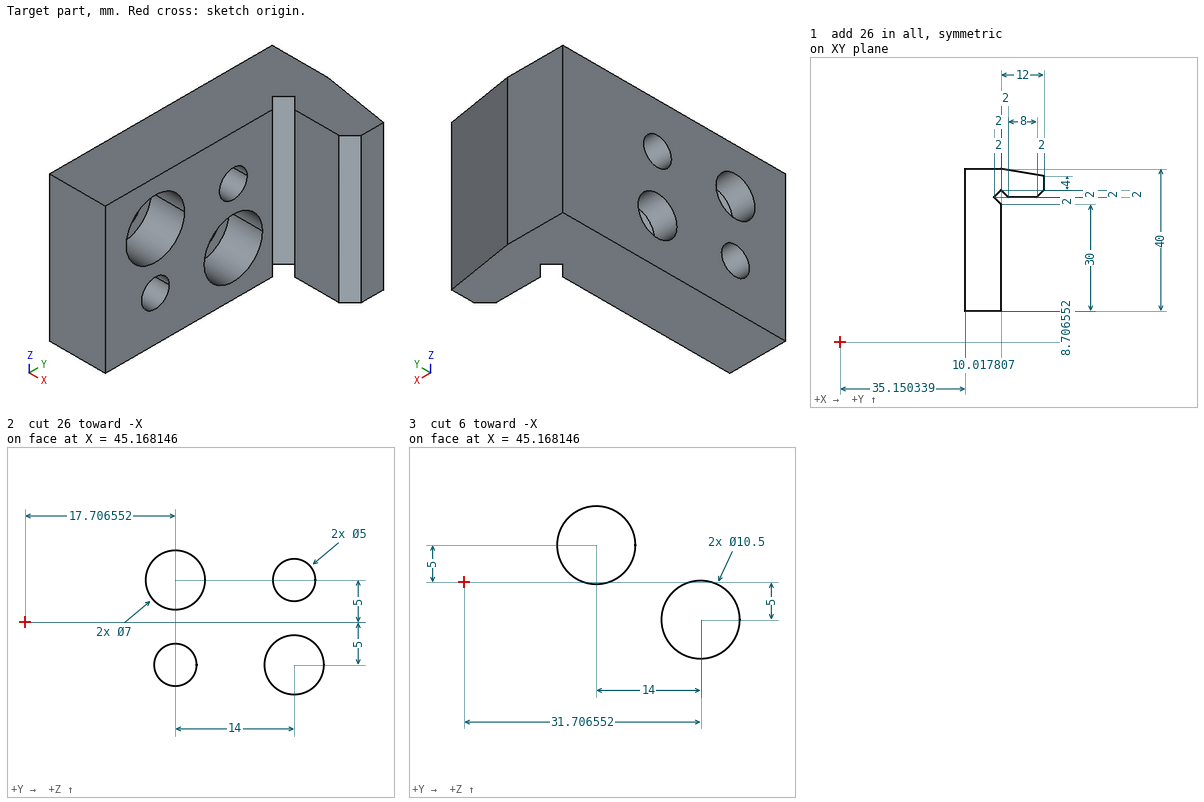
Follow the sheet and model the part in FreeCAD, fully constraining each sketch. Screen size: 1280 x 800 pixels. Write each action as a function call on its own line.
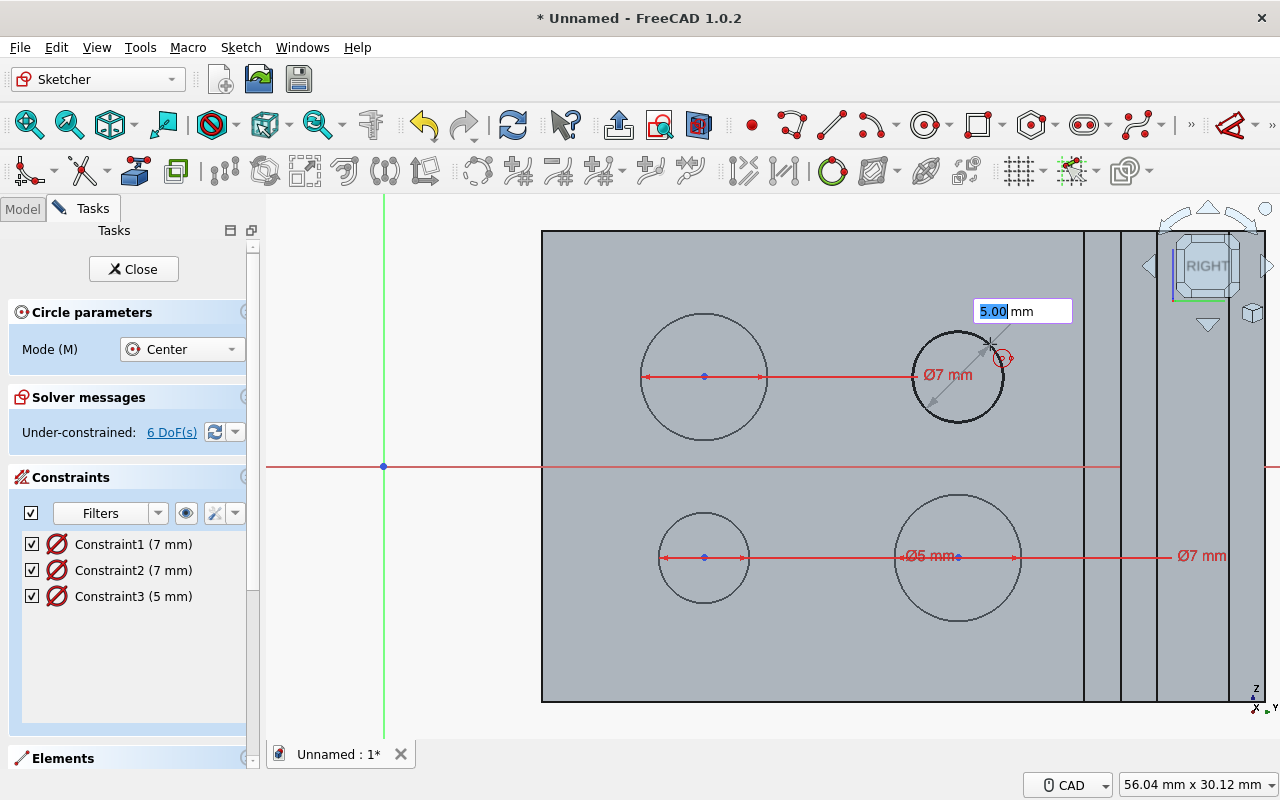
text(5)
key(Return)
key(Escape)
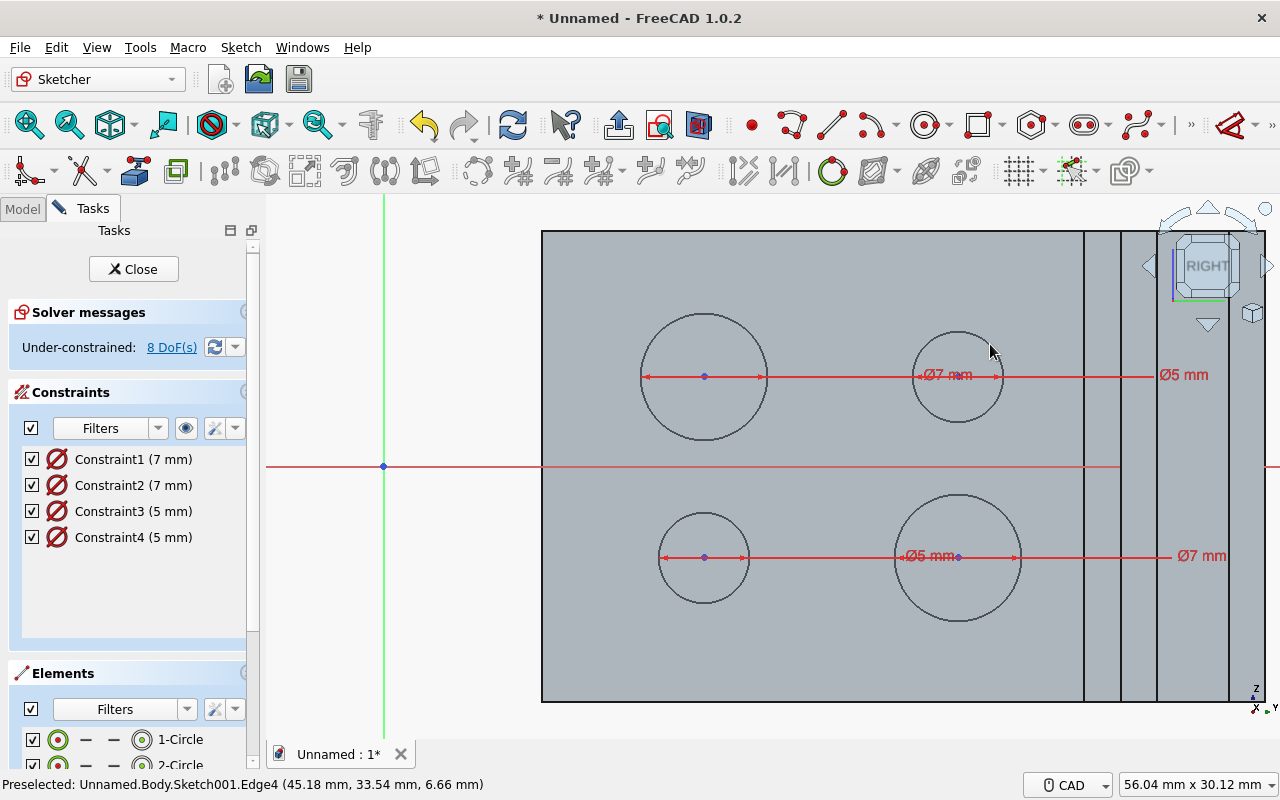
click(704, 377)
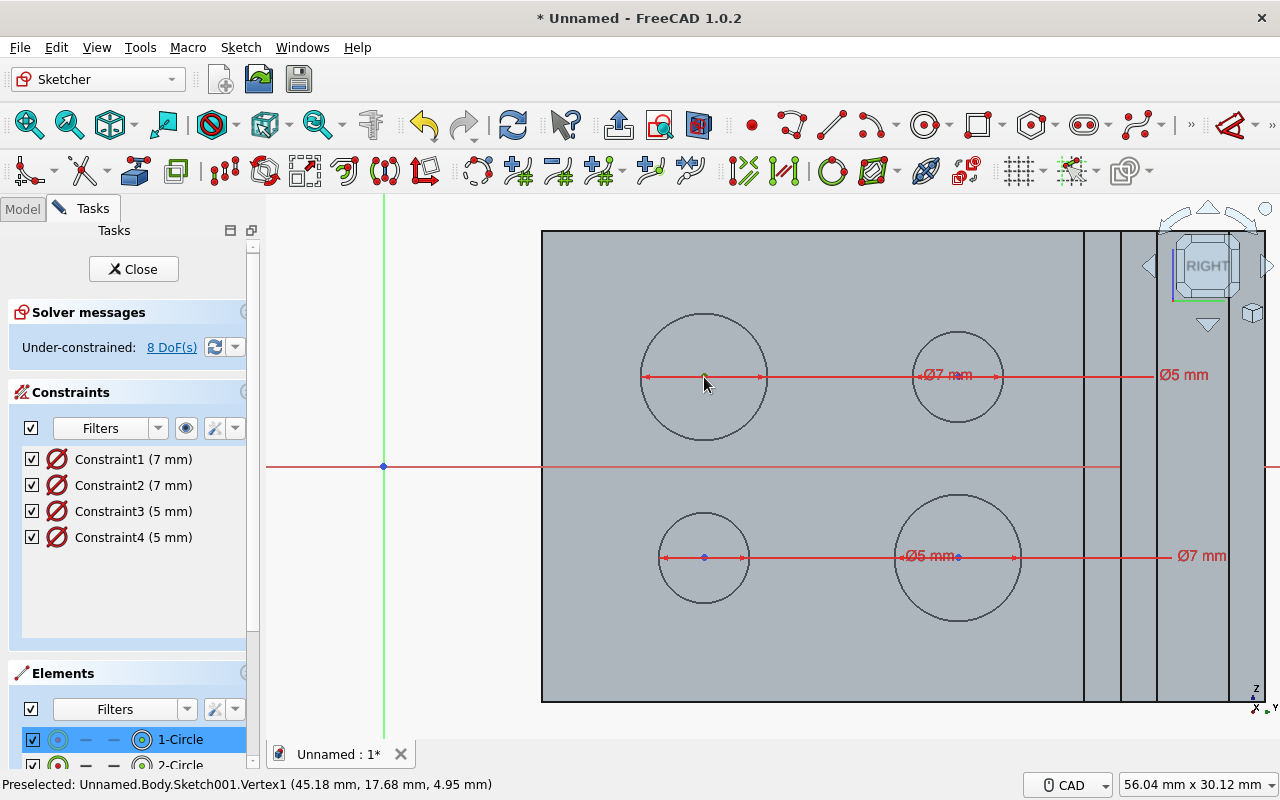
click(704, 558)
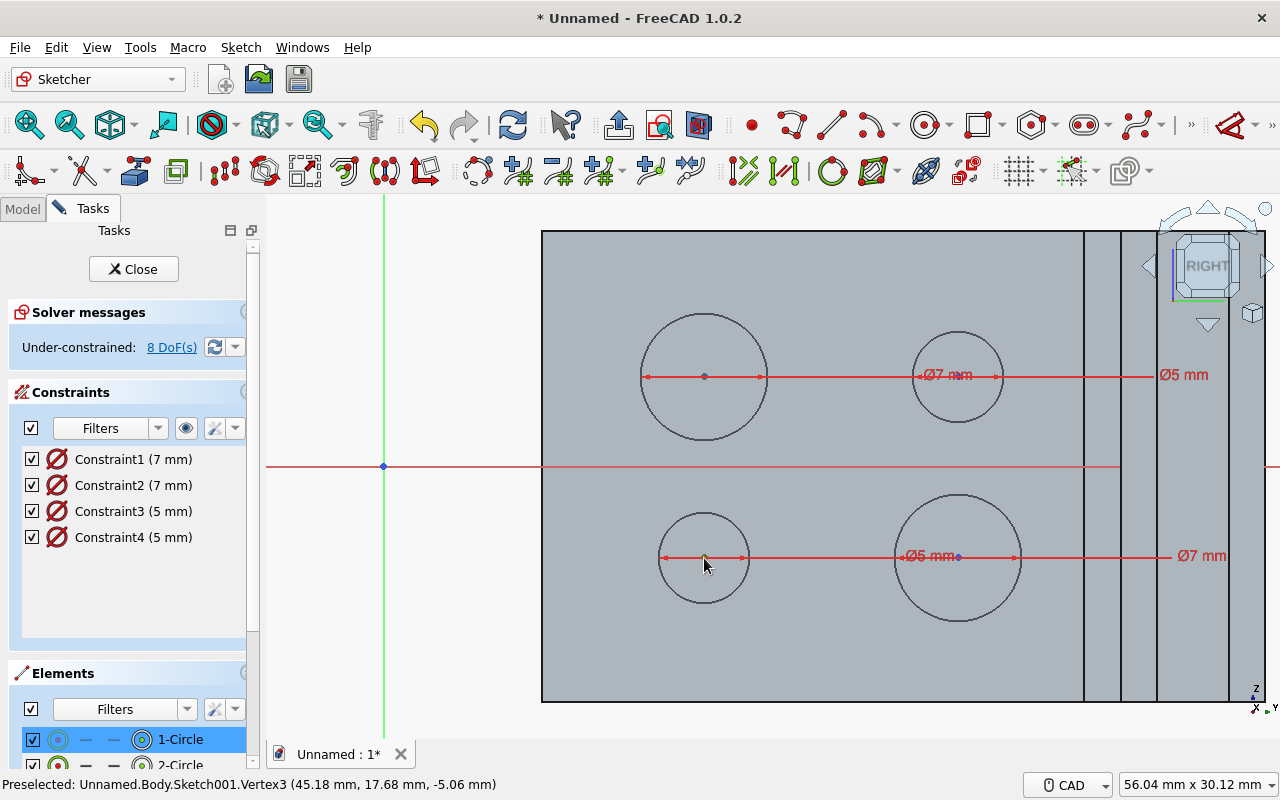
key(v)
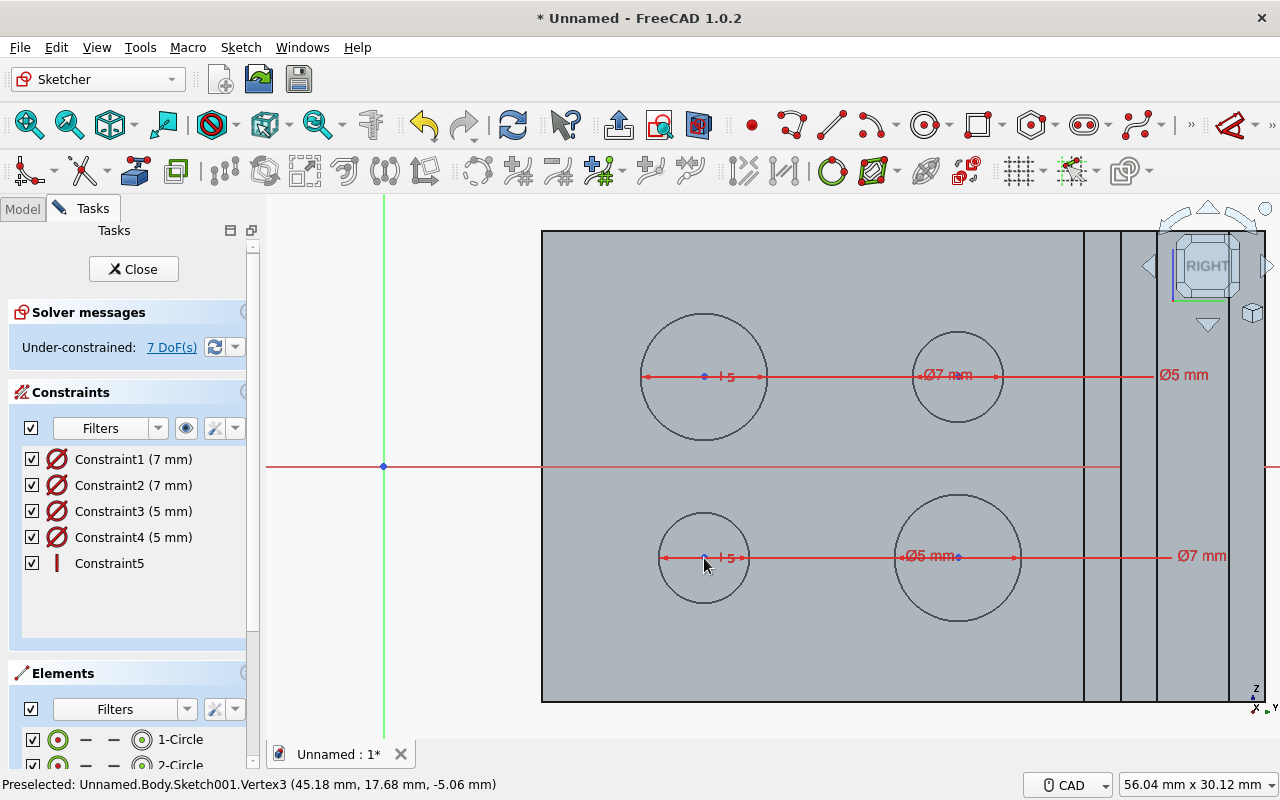
click(958, 558)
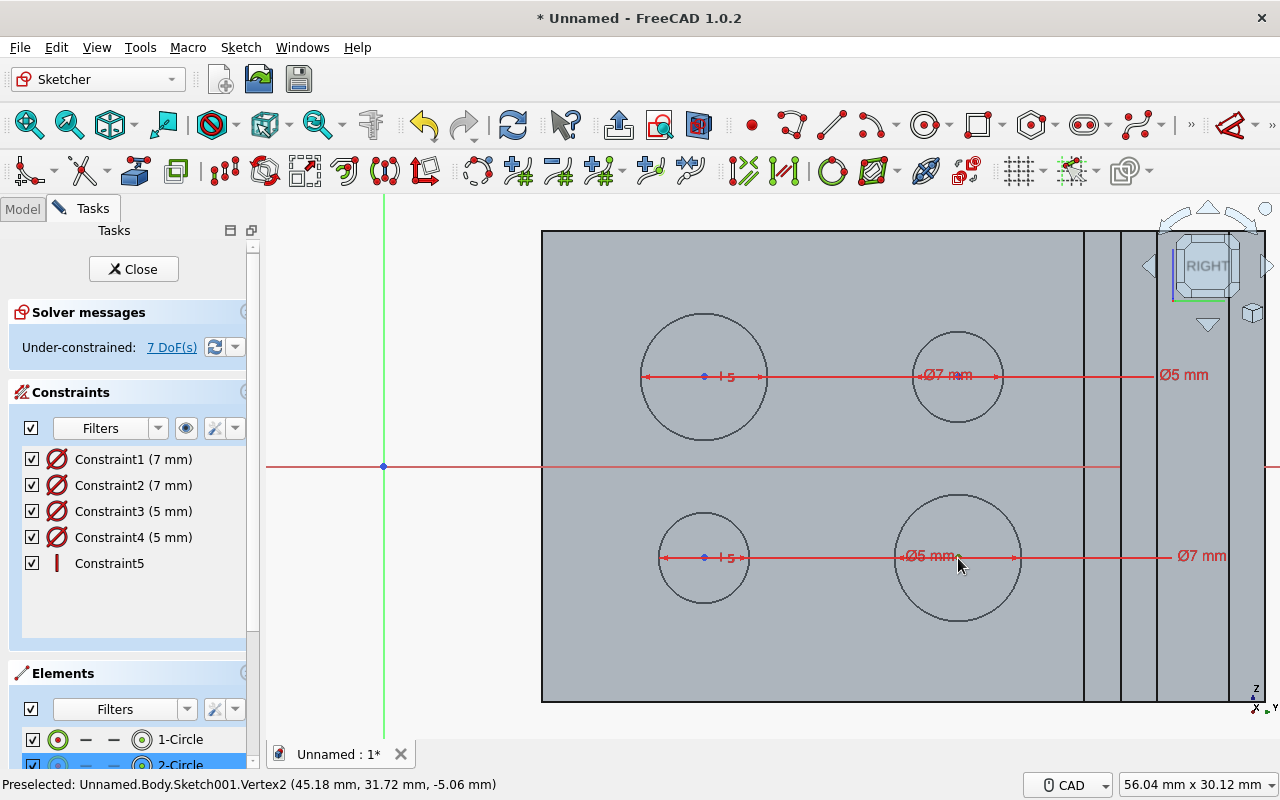
click(704, 558)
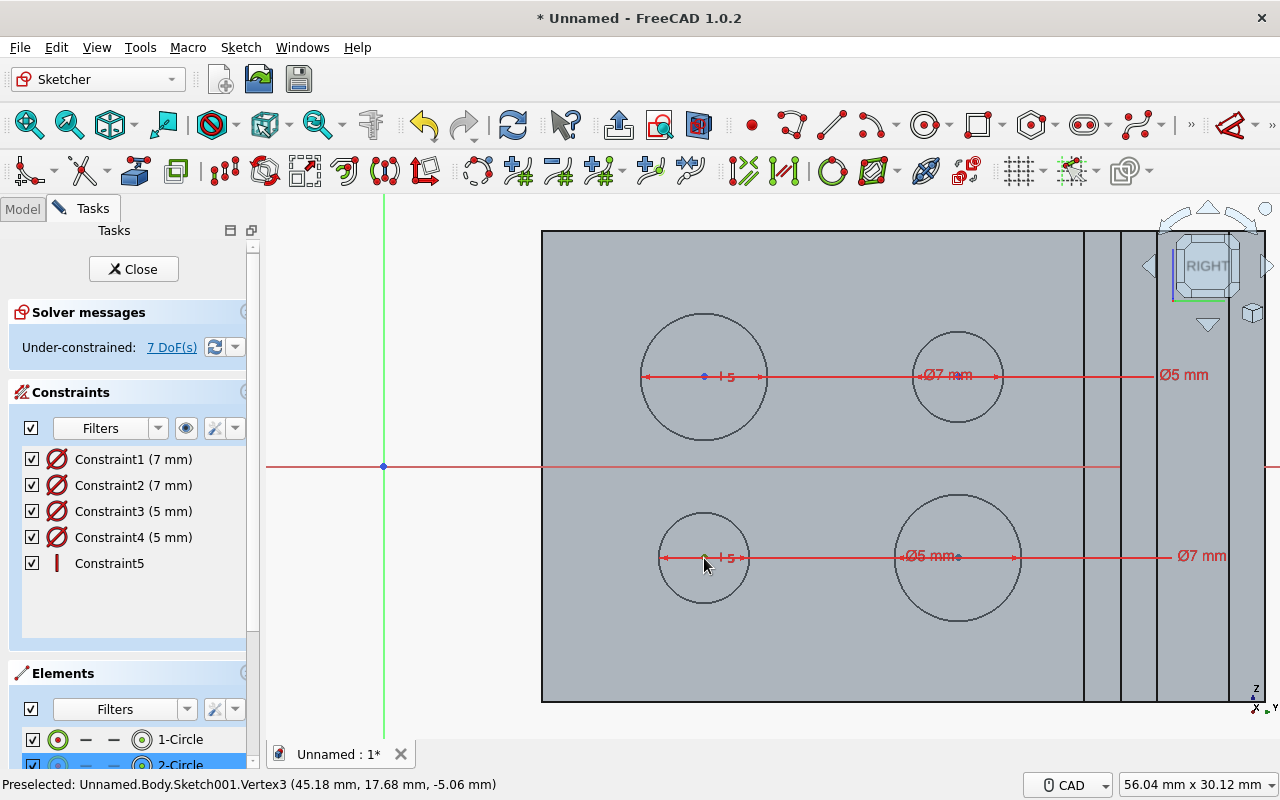
key(h)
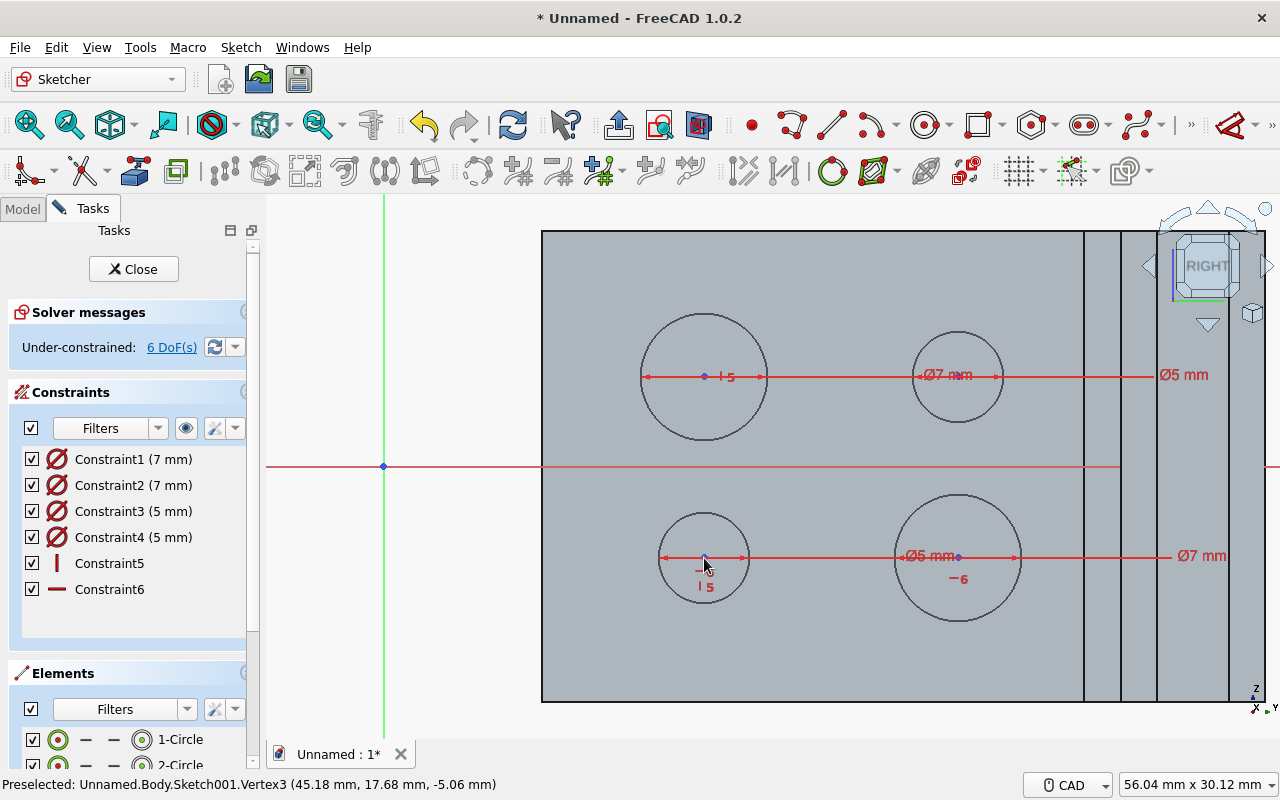
click(958, 558)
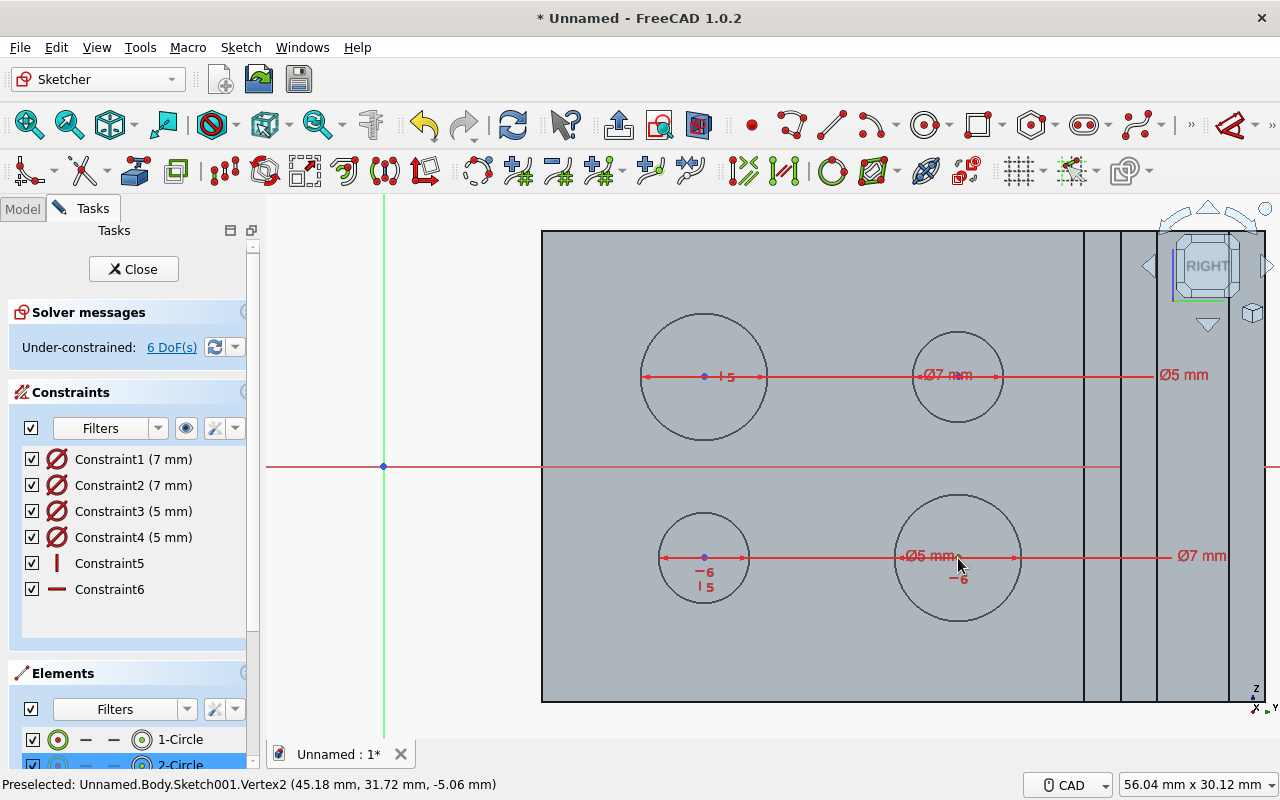
click(958, 377)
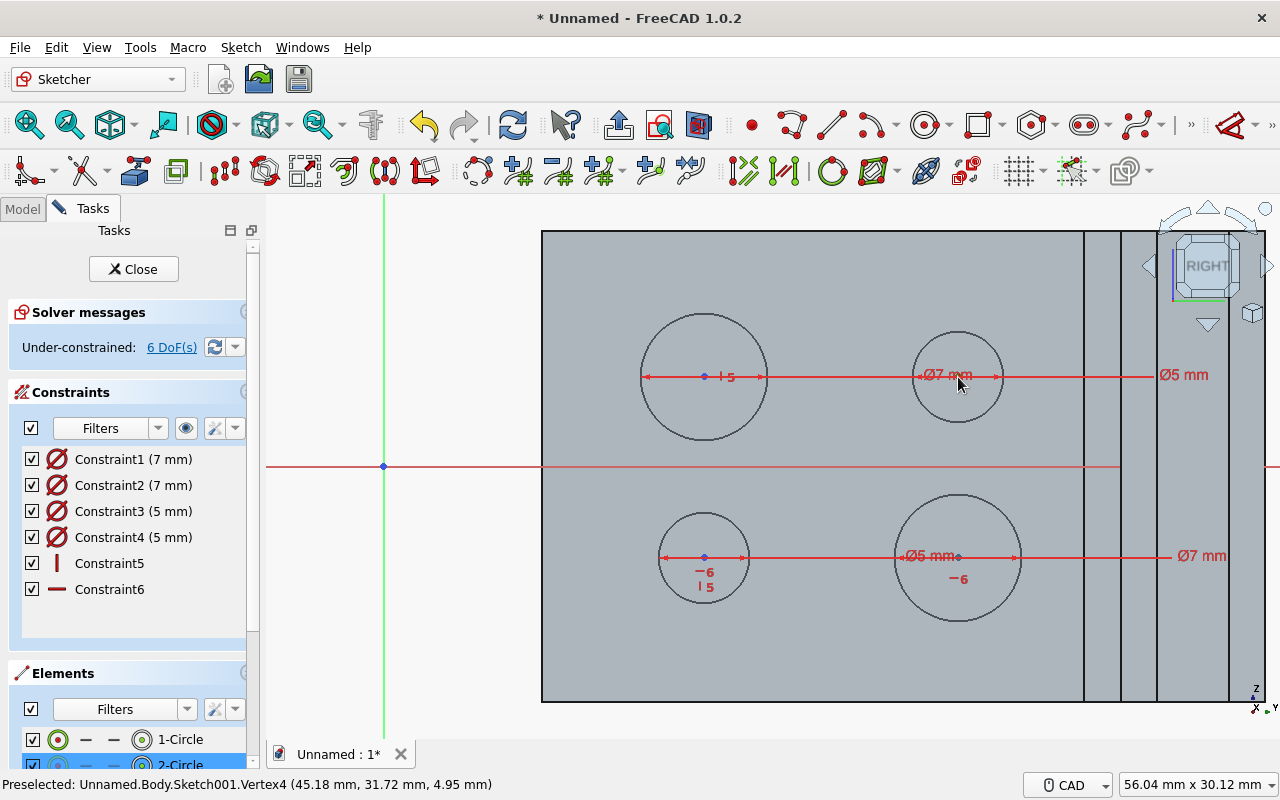
key(v)